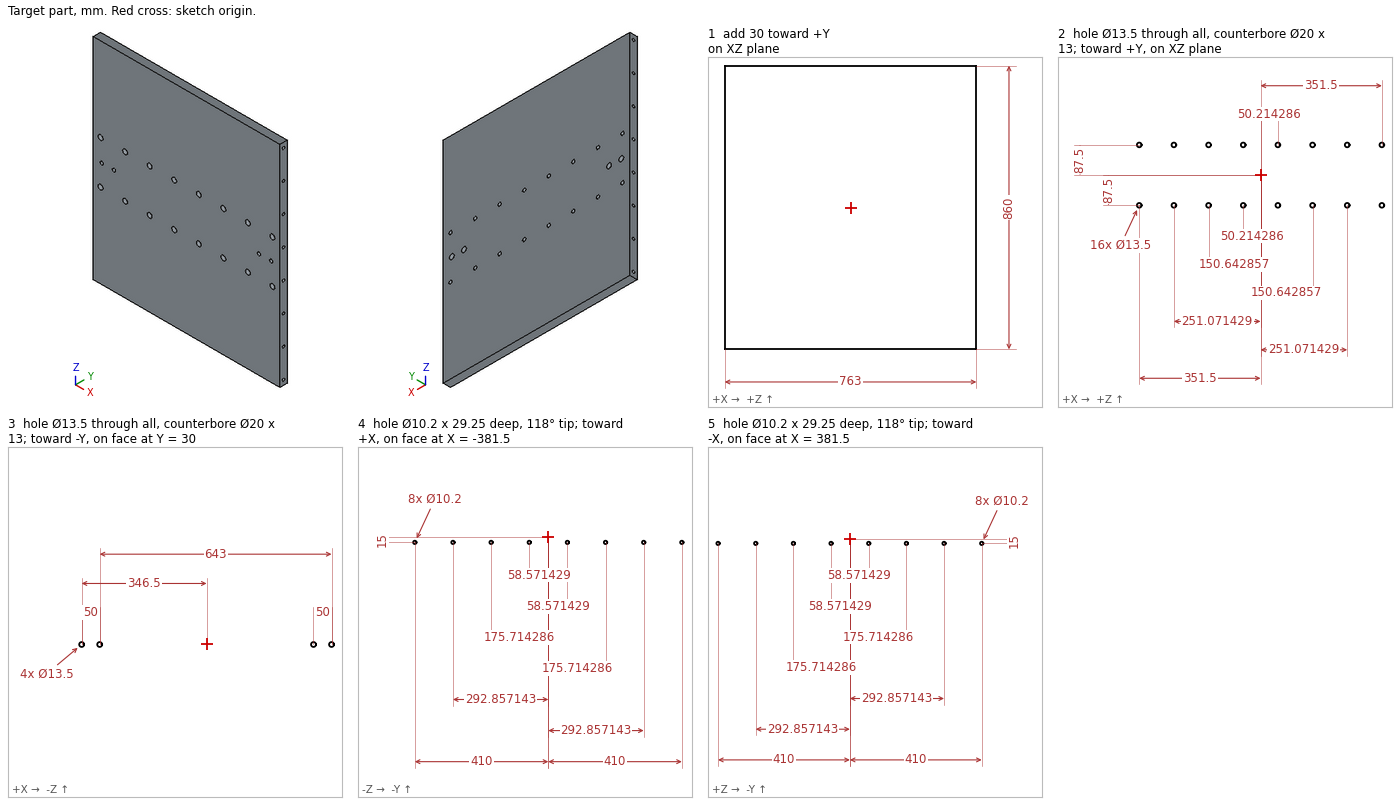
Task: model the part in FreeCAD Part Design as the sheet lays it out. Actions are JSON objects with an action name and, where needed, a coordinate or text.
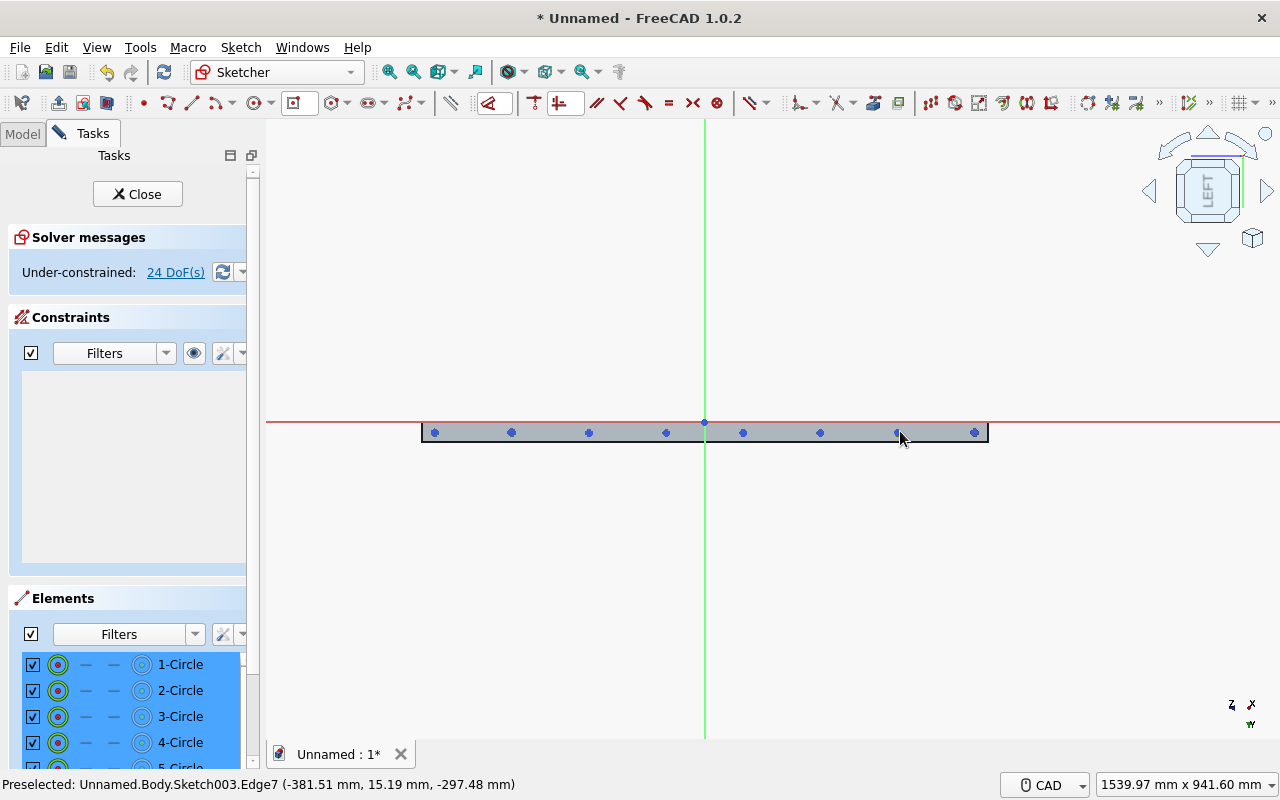
{"action": "scroll", "coordinate": [977, 430], "scroll_direction": "up", "scroll_amount": 8}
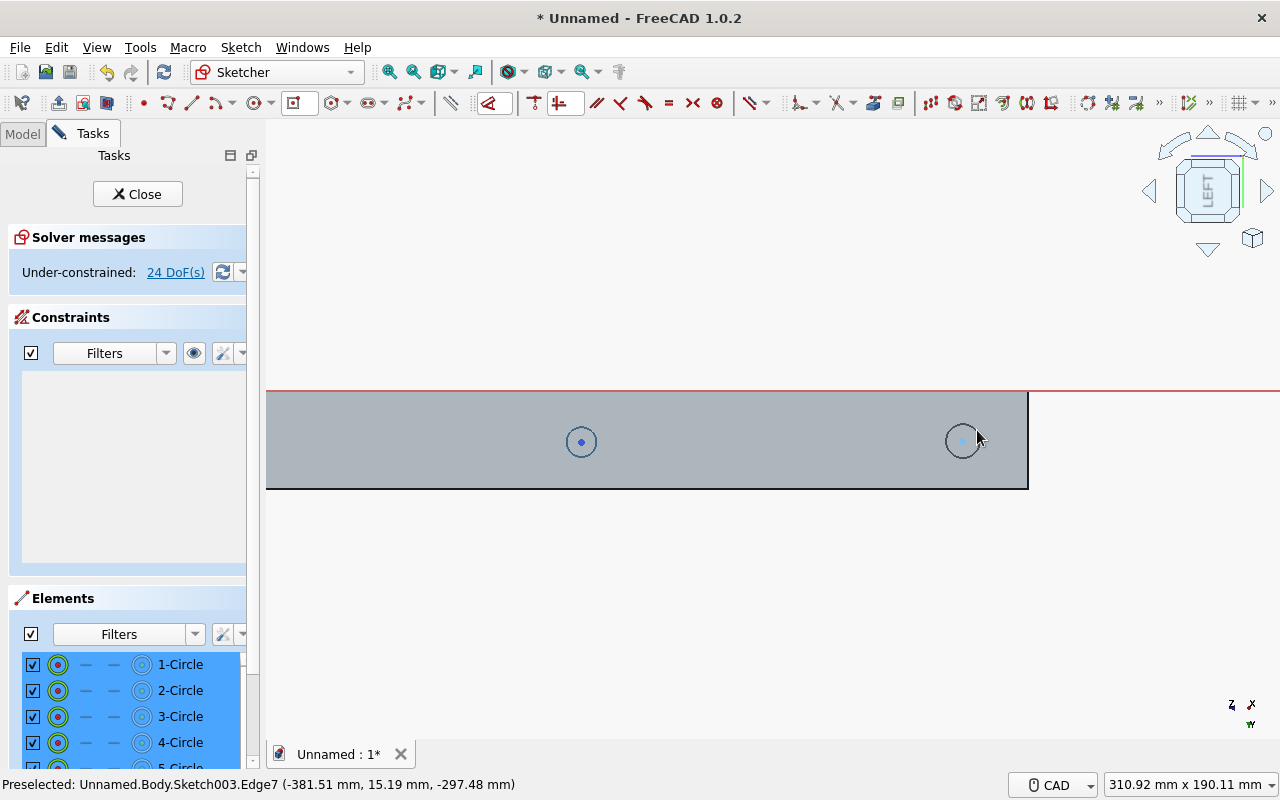
{"action": "left_click", "coordinate": [975, 429]}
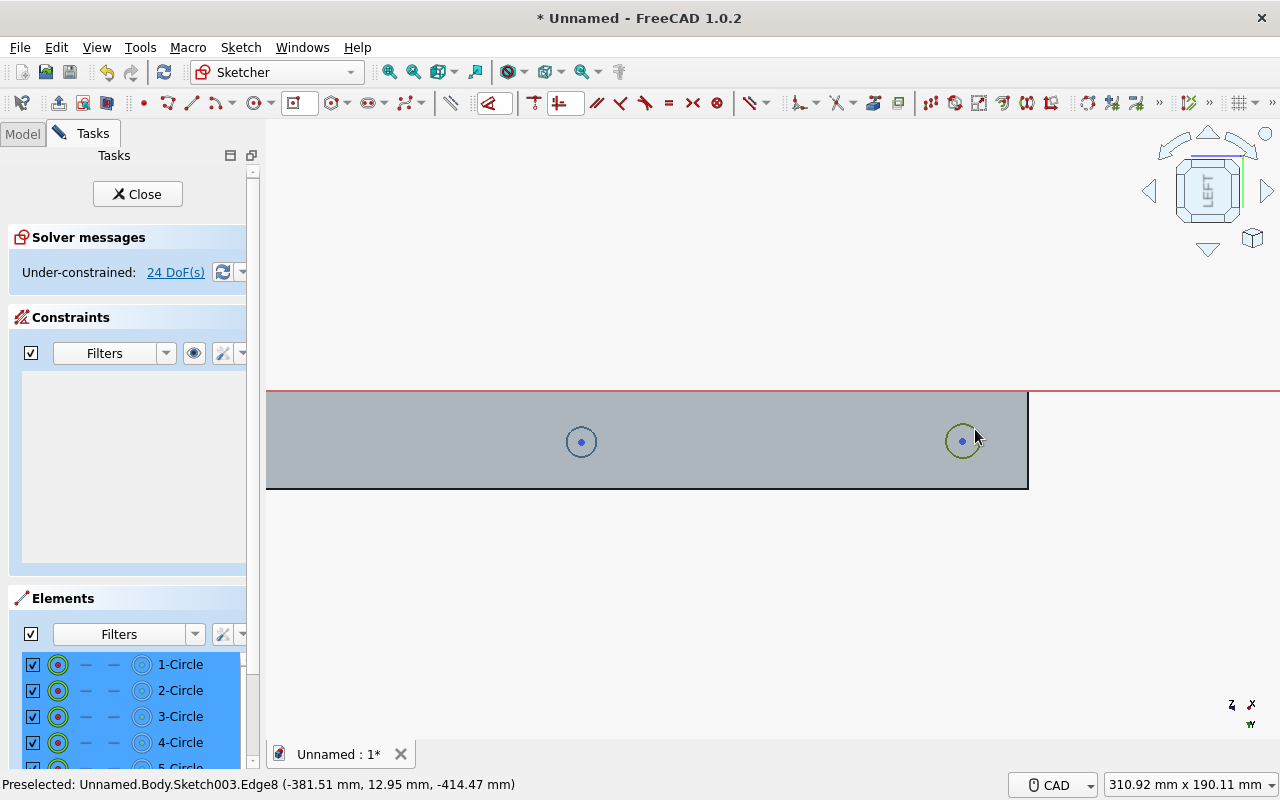
{"action": "left_click", "coordinate": [670, 104]}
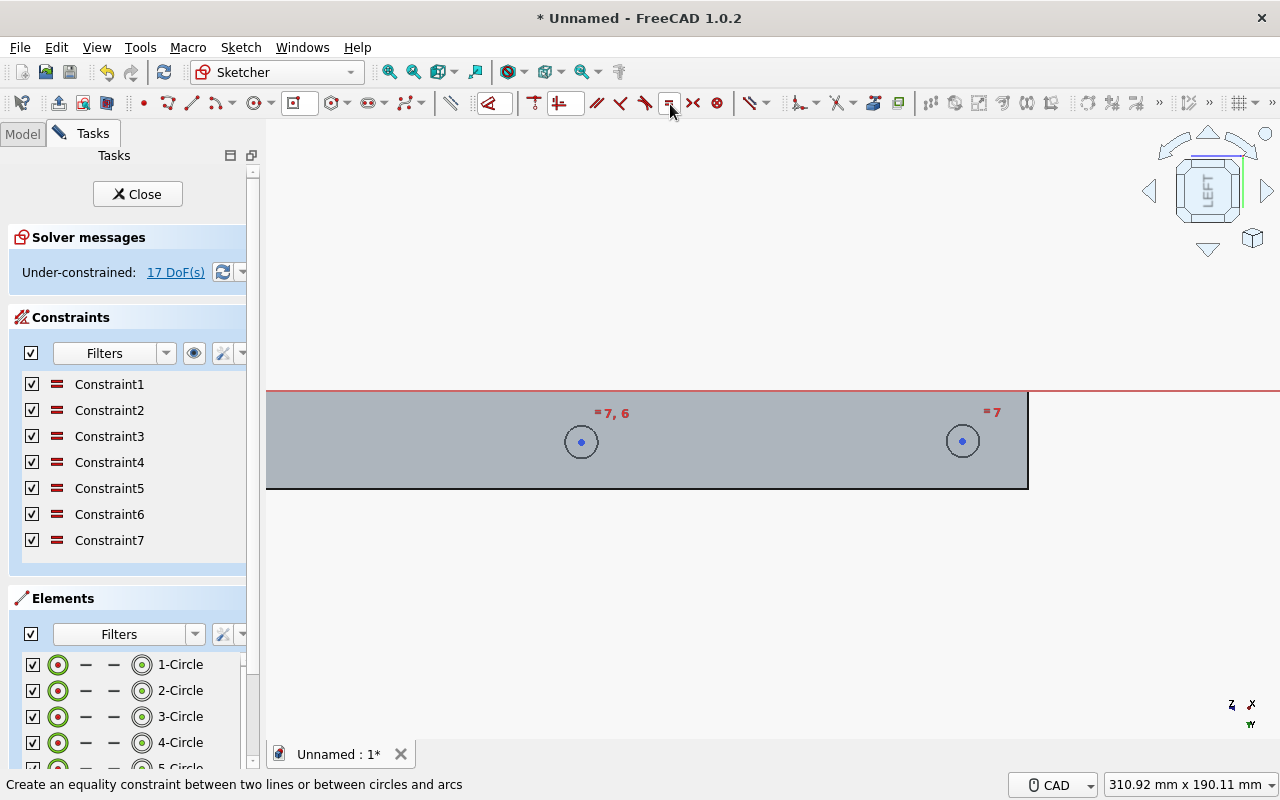
{"action": "scroll", "coordinate": [977, 430], "scroll_direction": "down", "scroll_amount": 8}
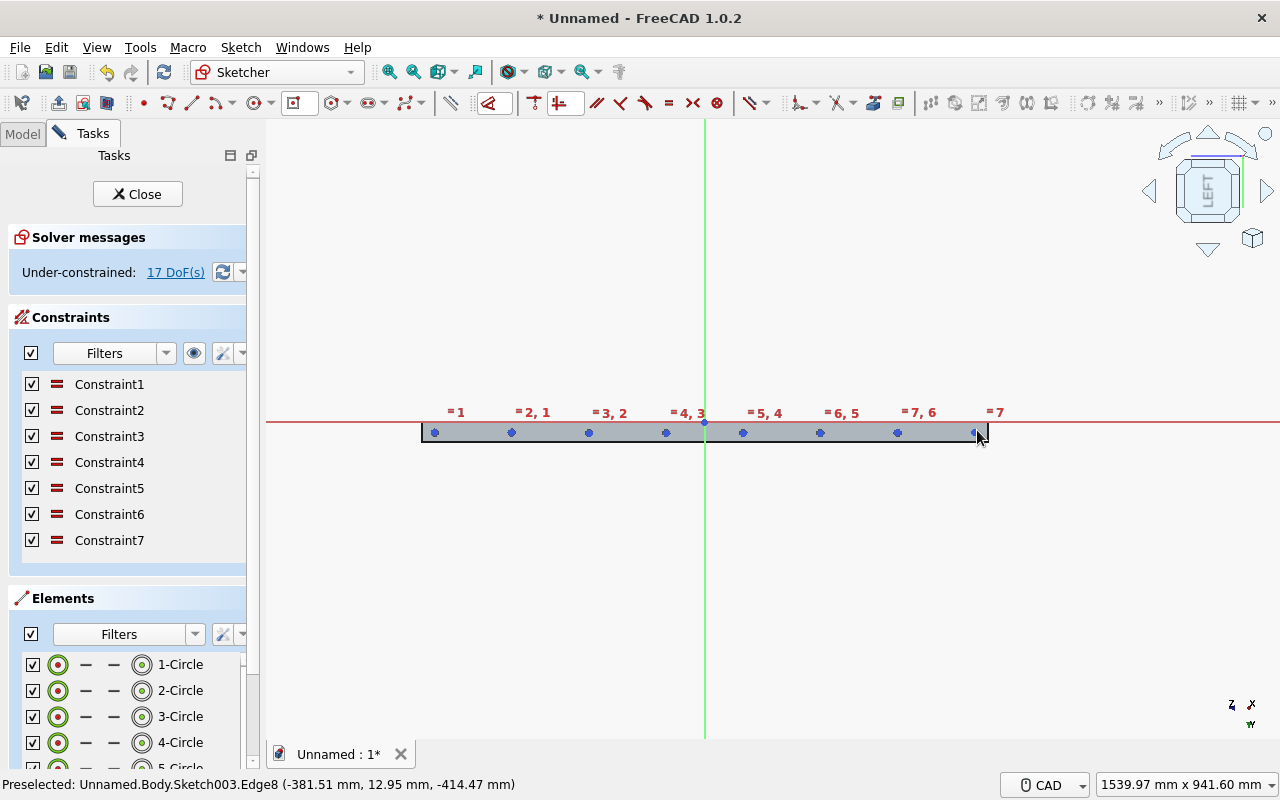
{"action": "left_click", "coordinate": [435, 433]}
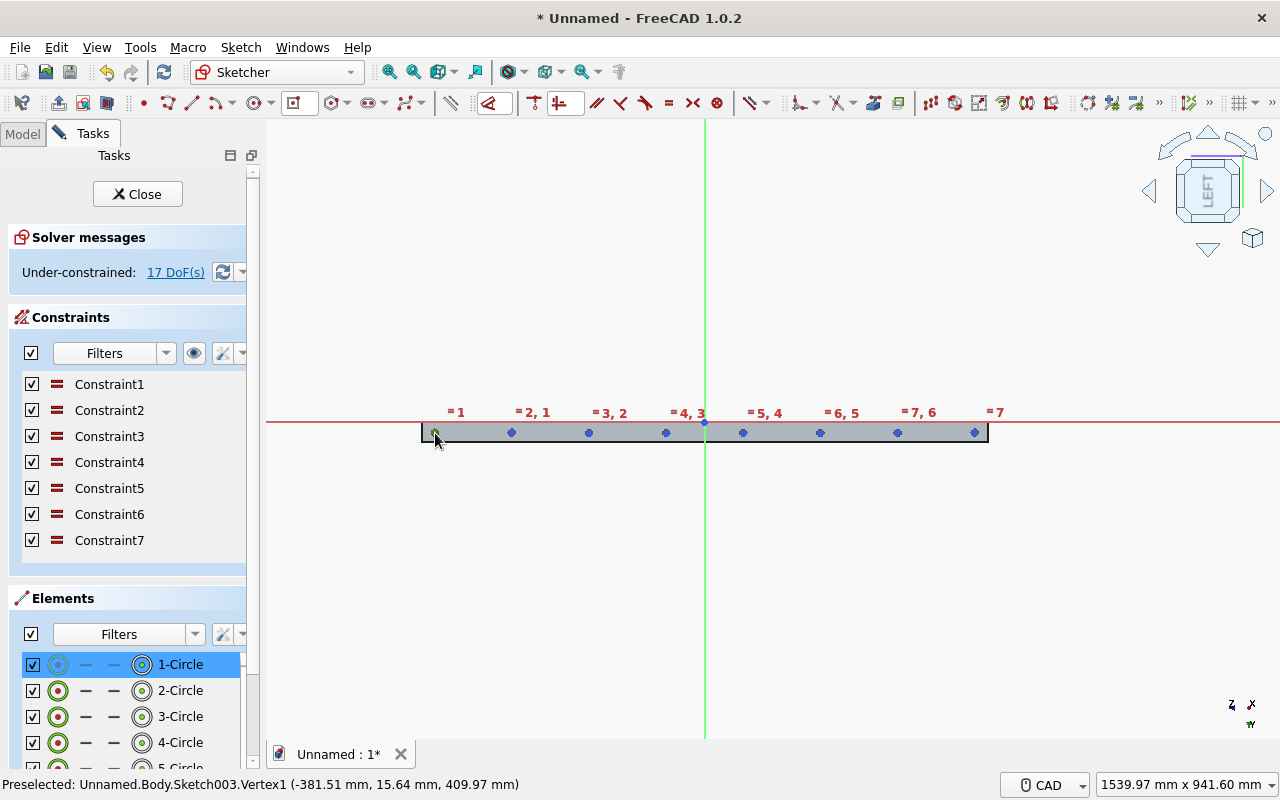
{"action": "left_click", "coordinate": [512, 433]}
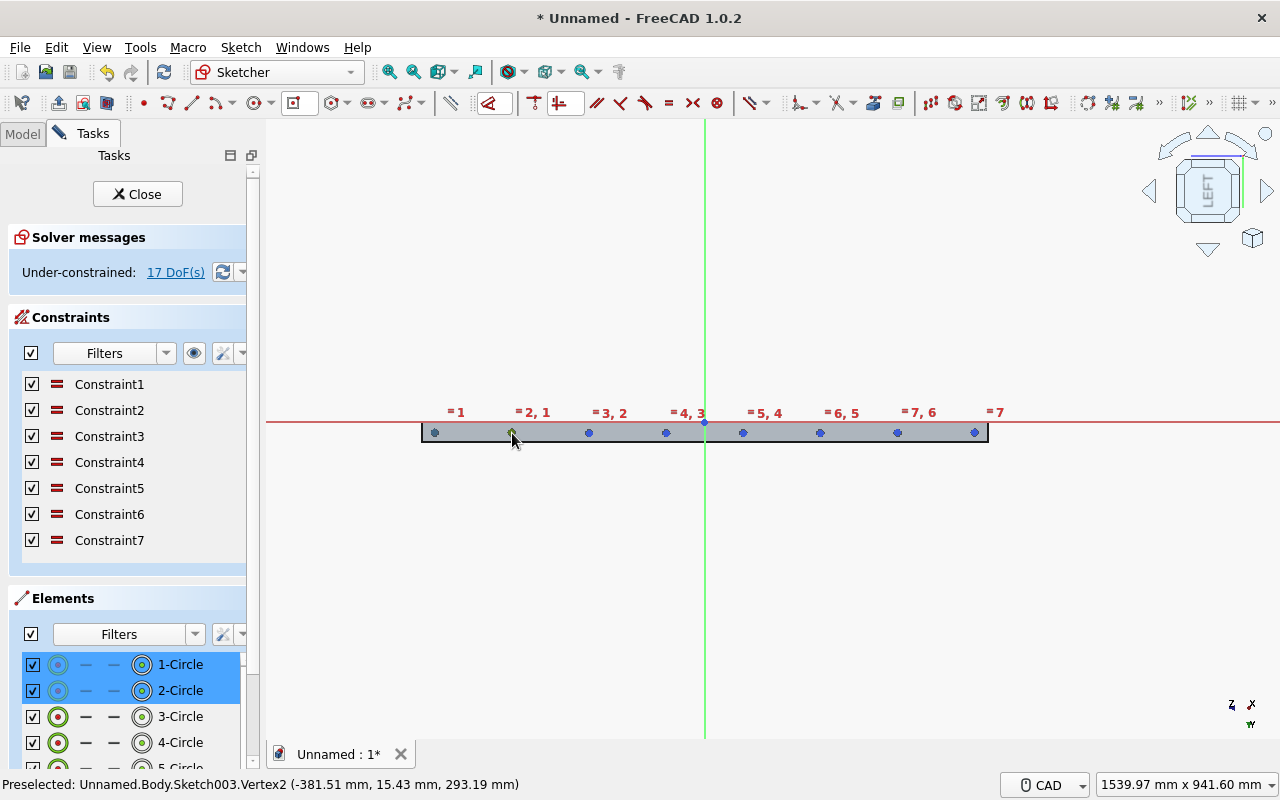
{"action": "key", "text": "h"}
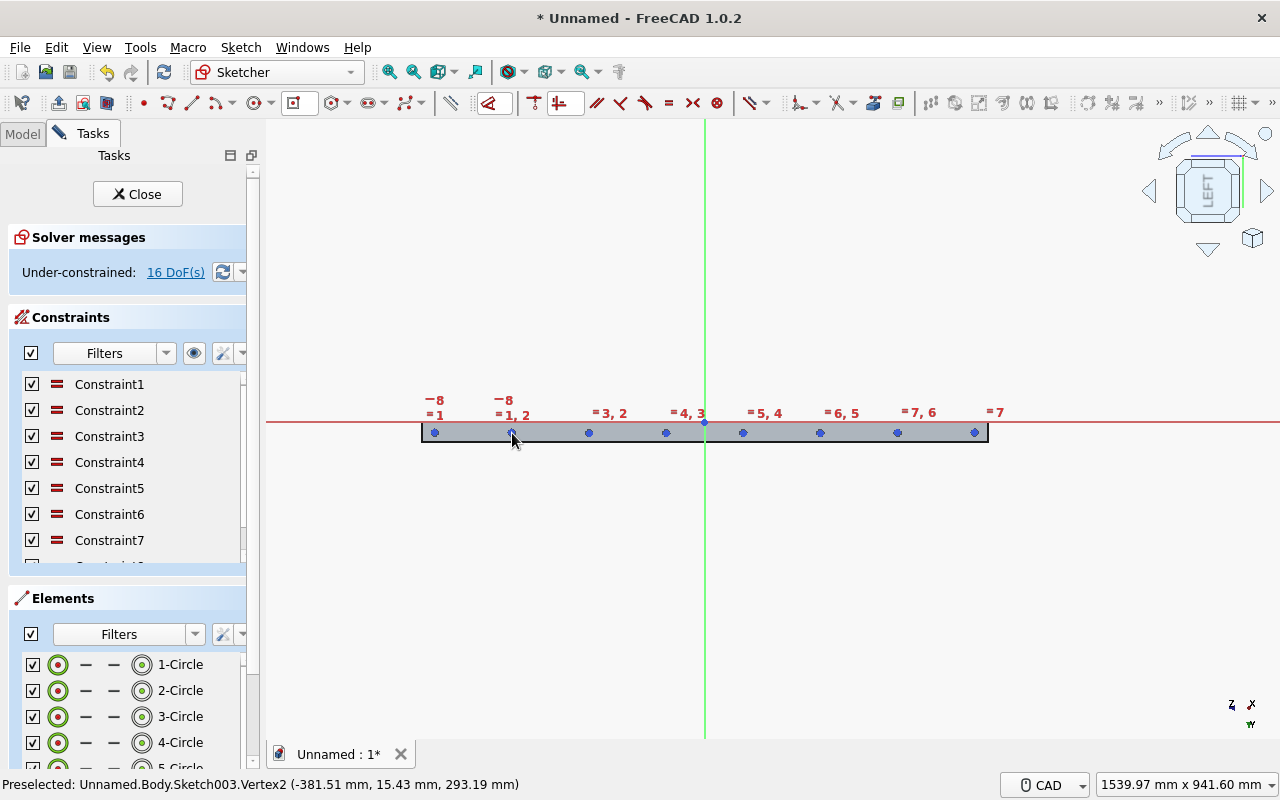
{"action": "left_click", "coordinate": [512, 433]}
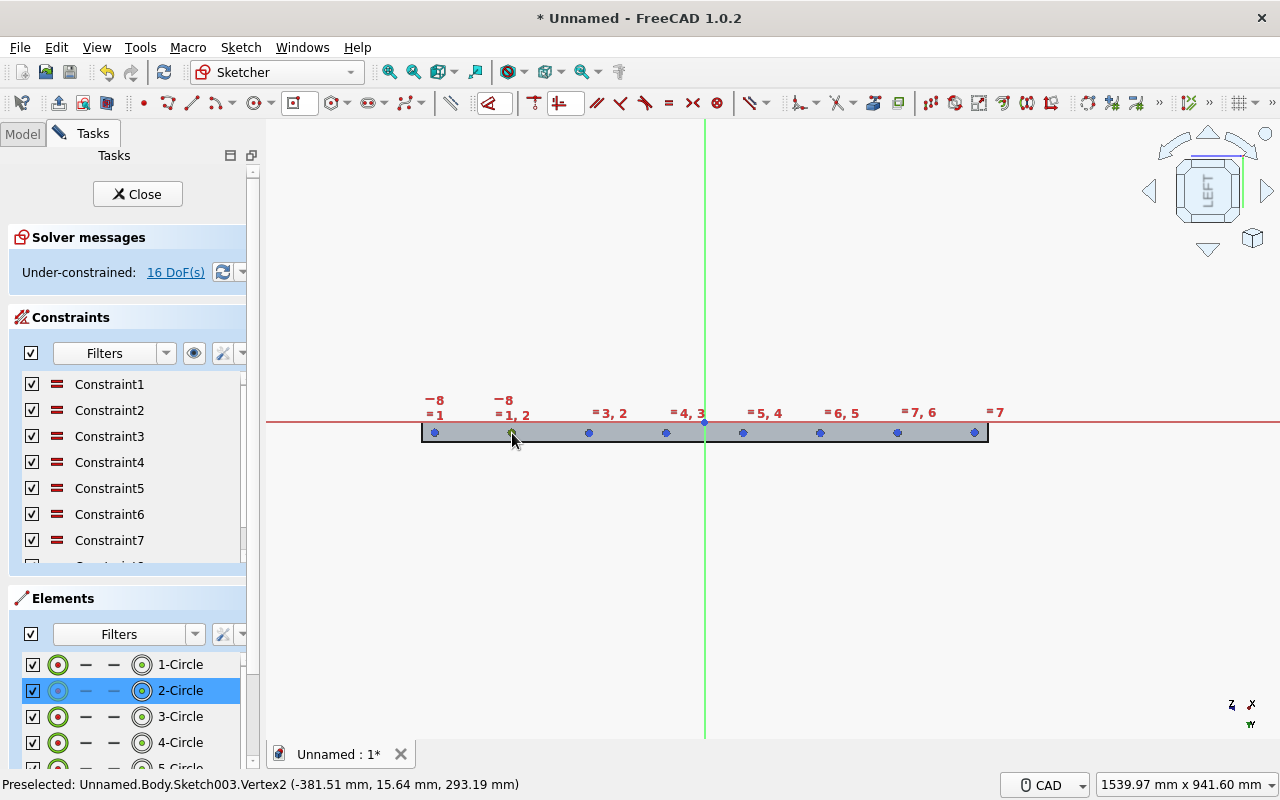
{"action": "left_click", "coordinate": [589, 433]}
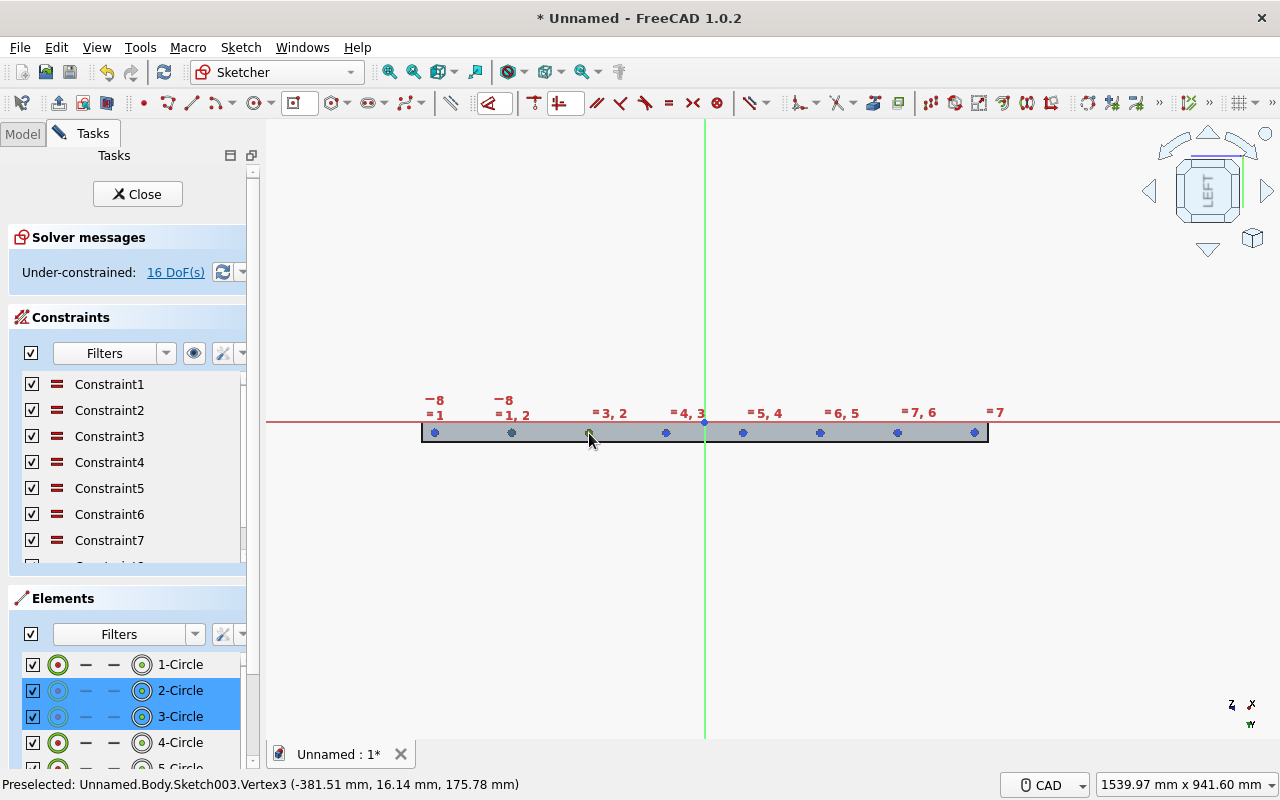
{"action": "key", "text": "h"}